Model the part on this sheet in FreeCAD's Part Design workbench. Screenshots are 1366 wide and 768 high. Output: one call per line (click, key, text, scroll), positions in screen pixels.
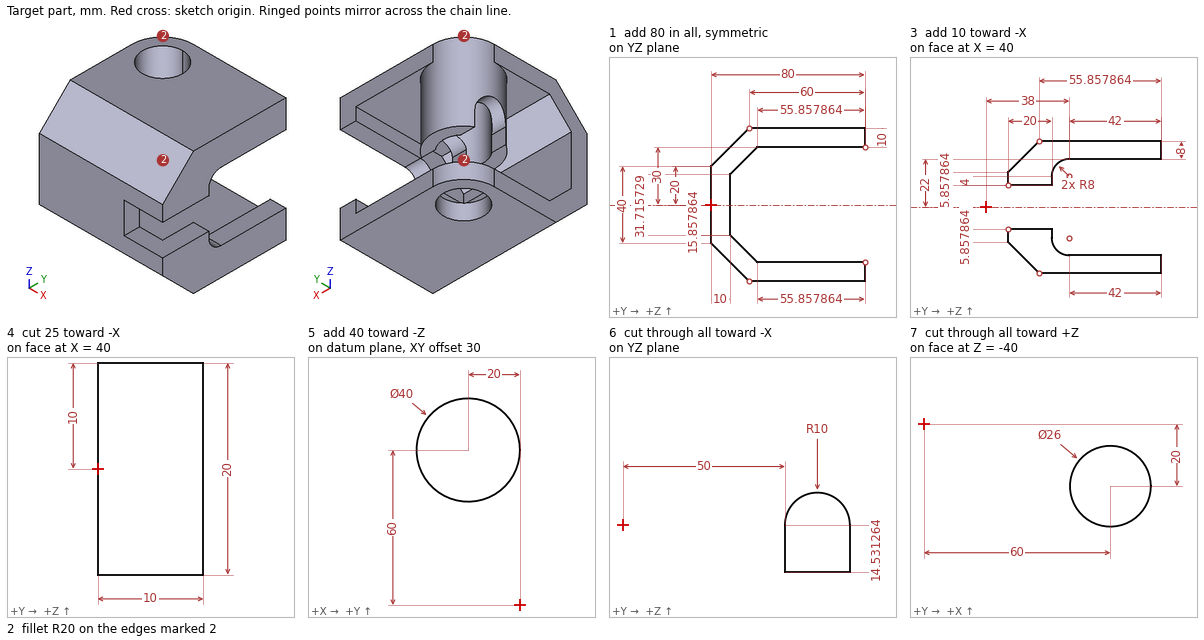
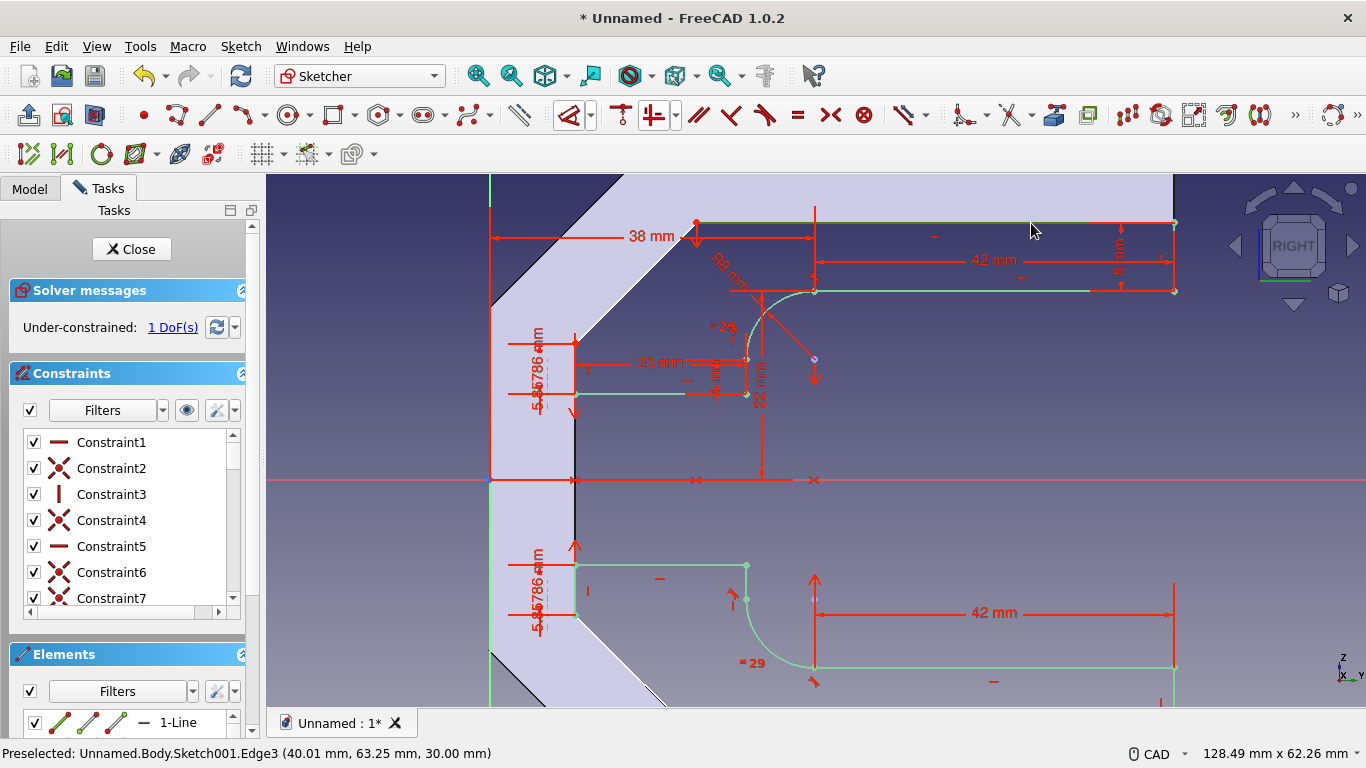
click(590, 116)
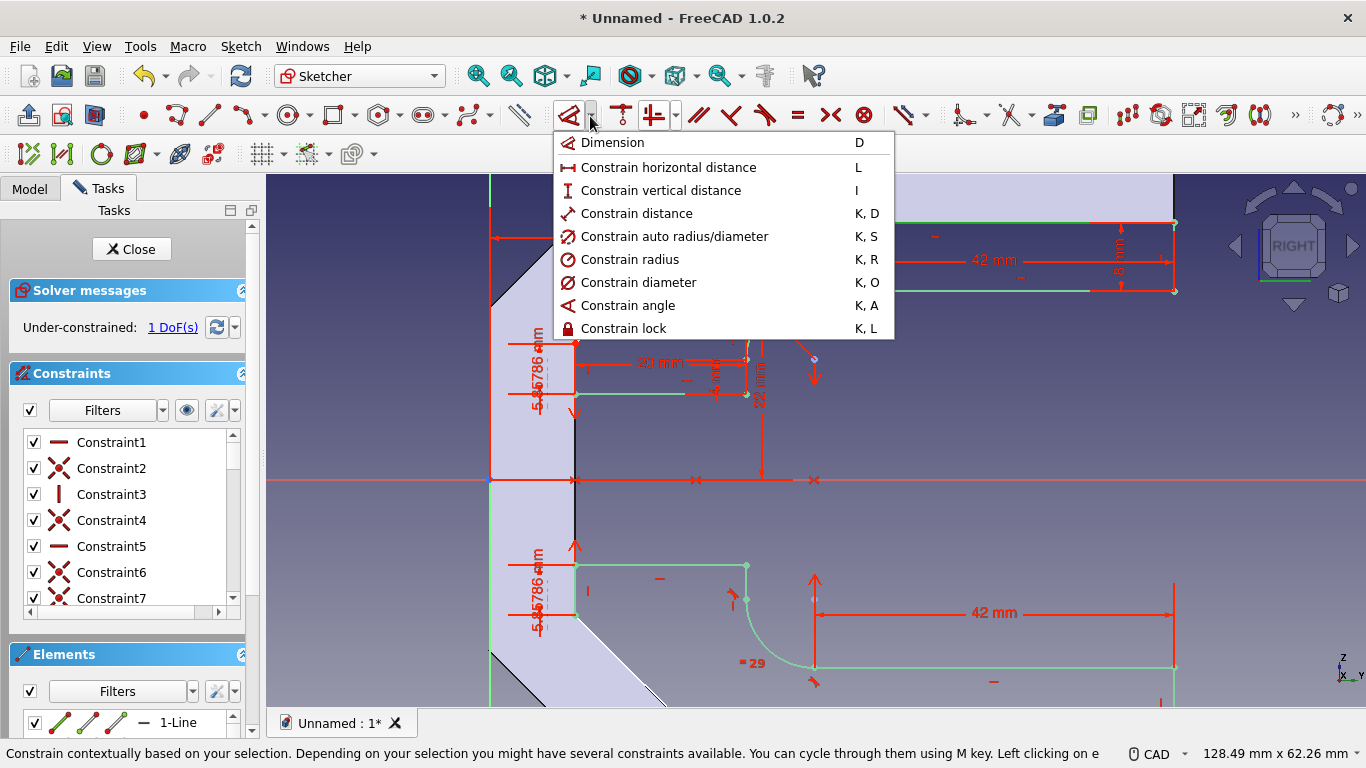
click(724, 168)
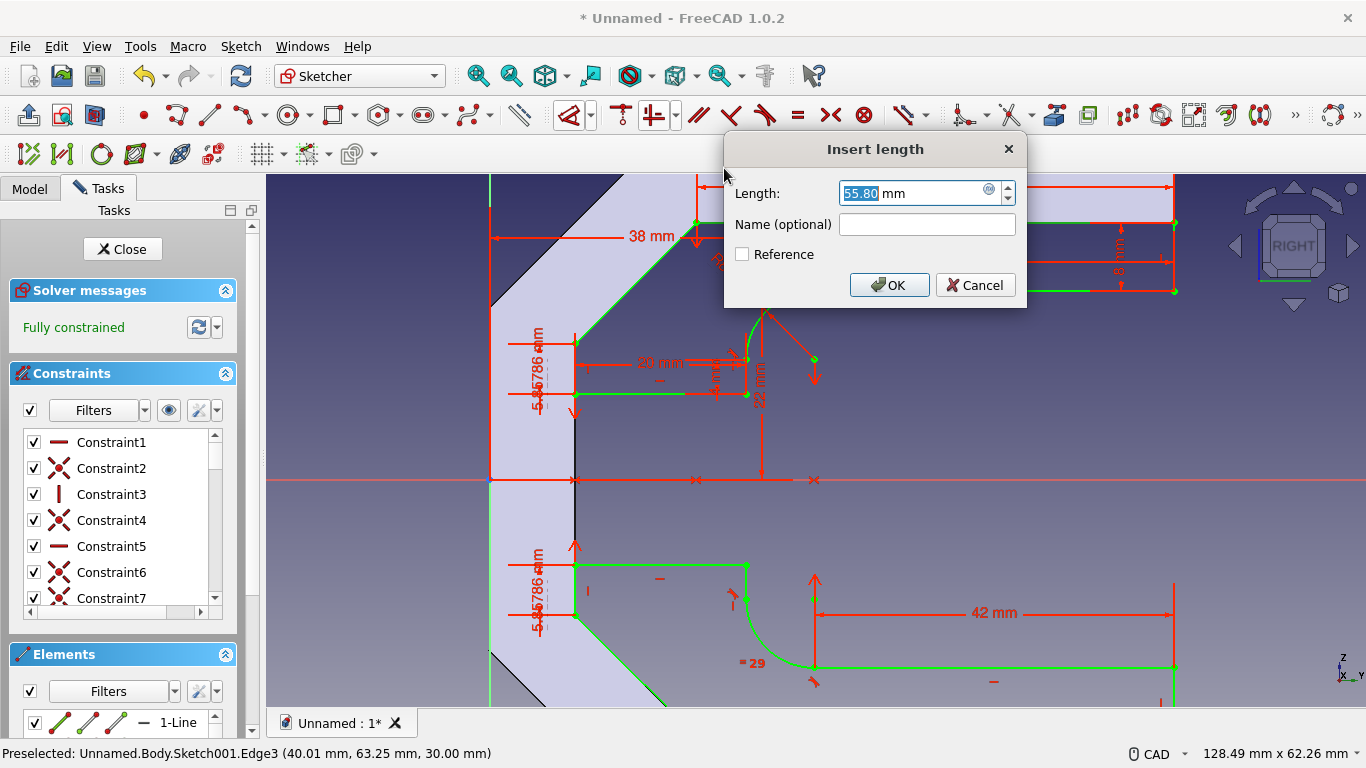
text(55.857864)
key(Return)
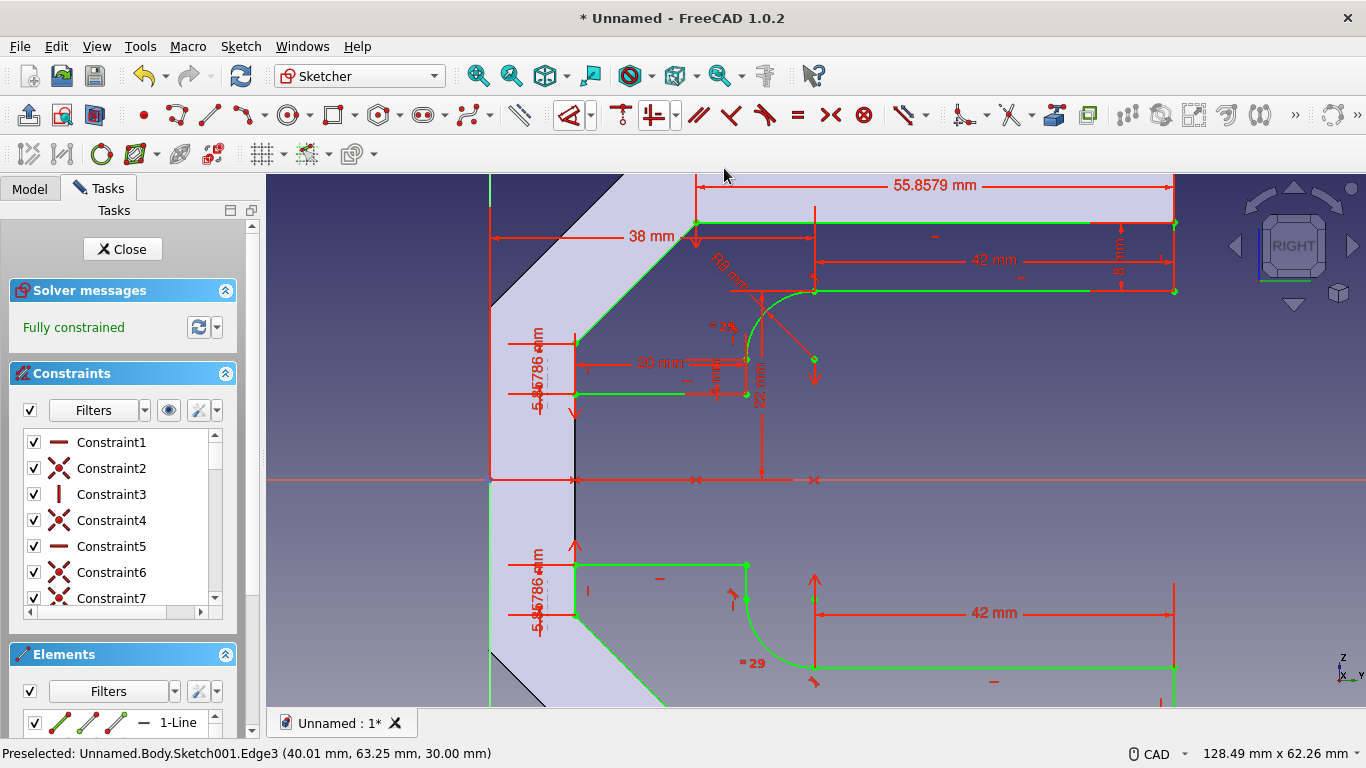
click(123, 249)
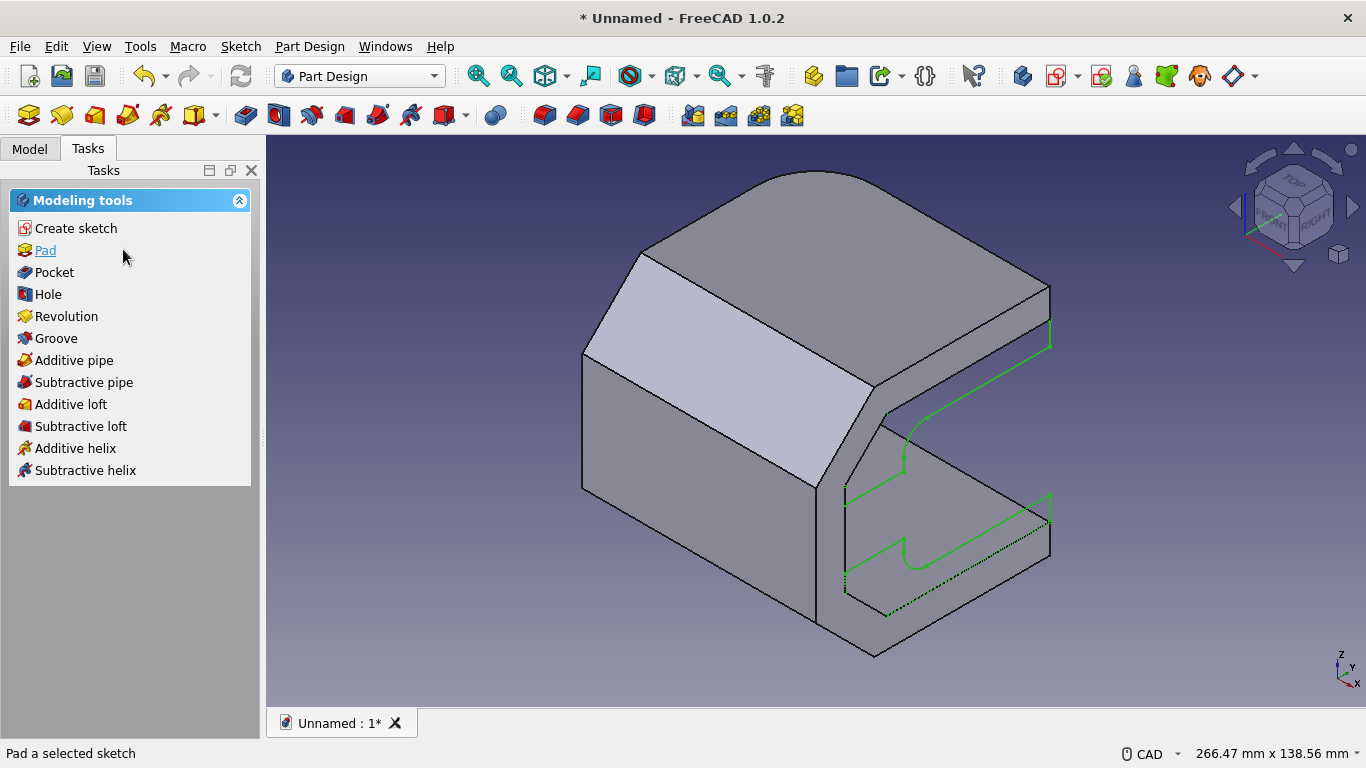
click(29, 116)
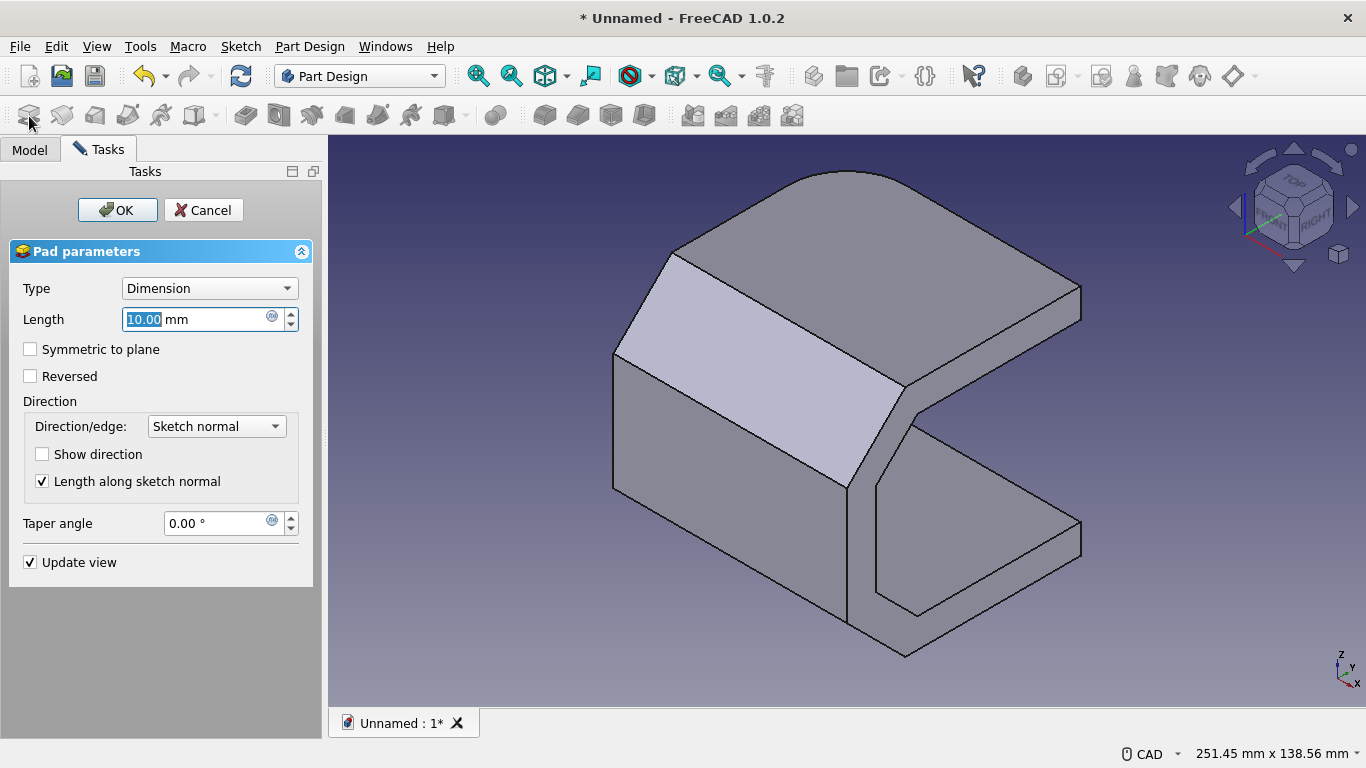
text(10)
key(Tab)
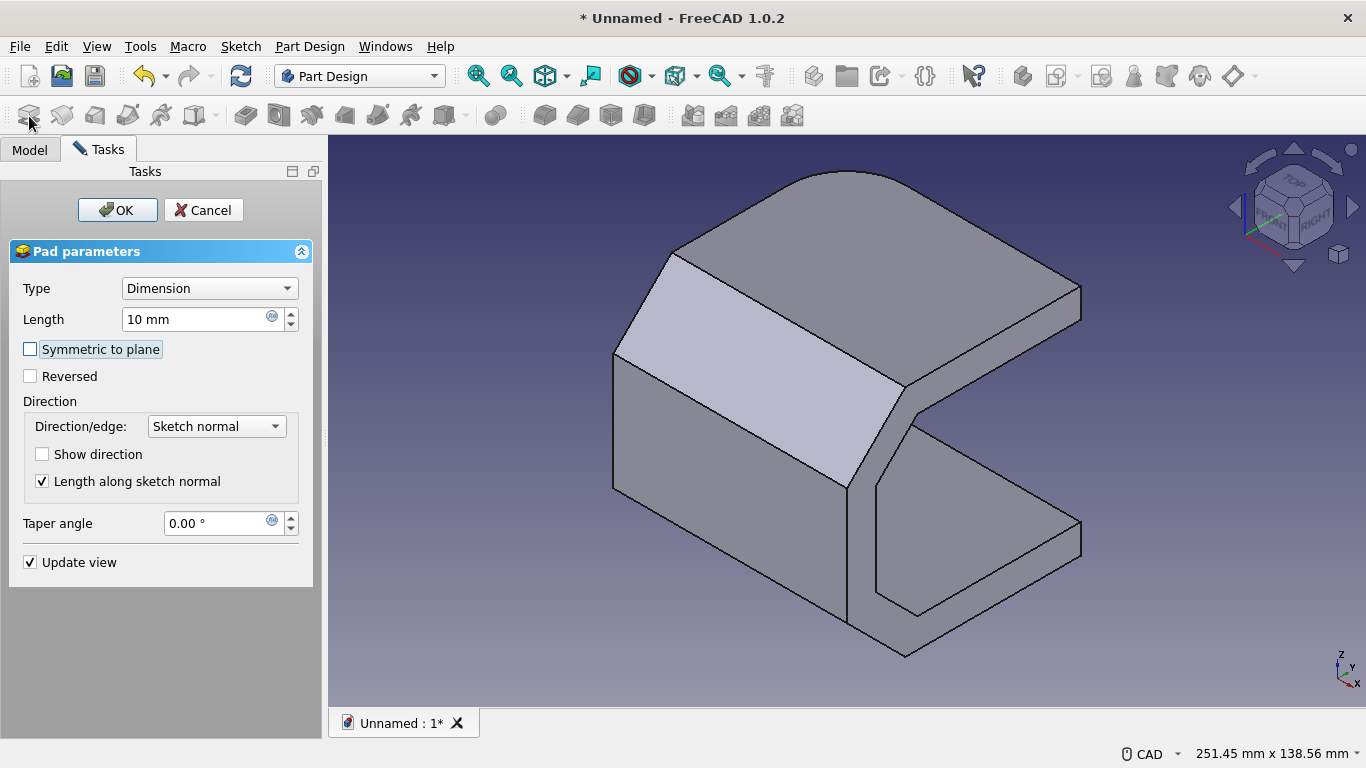
click(31, 376)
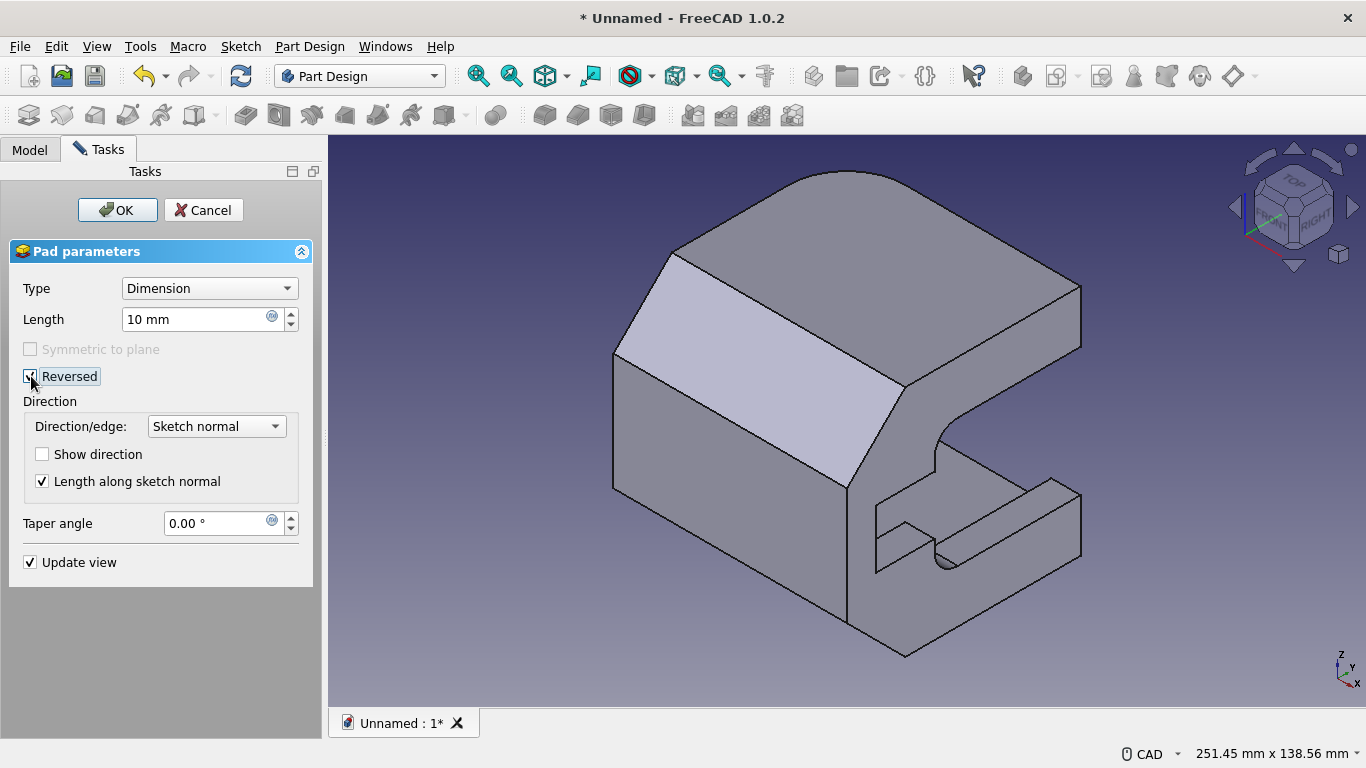
click(118, 210)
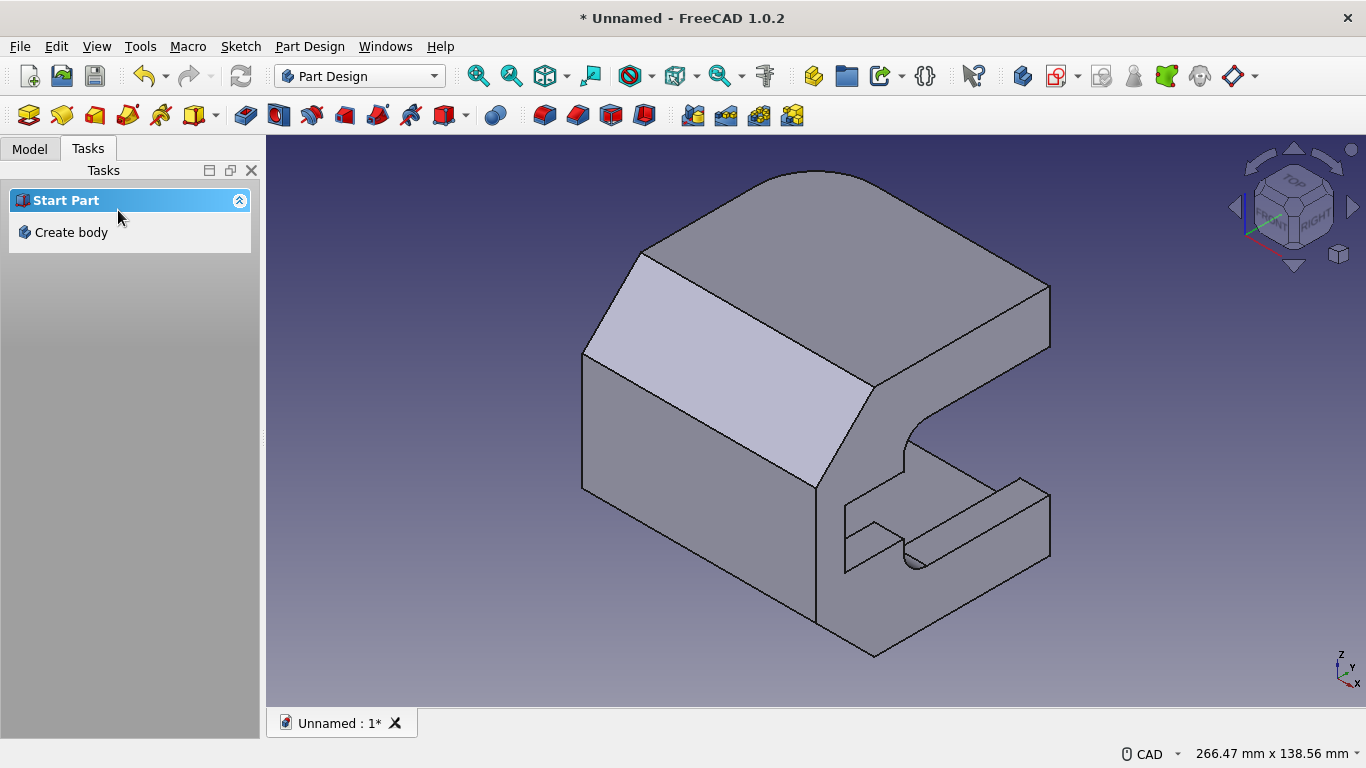
click(866, 449)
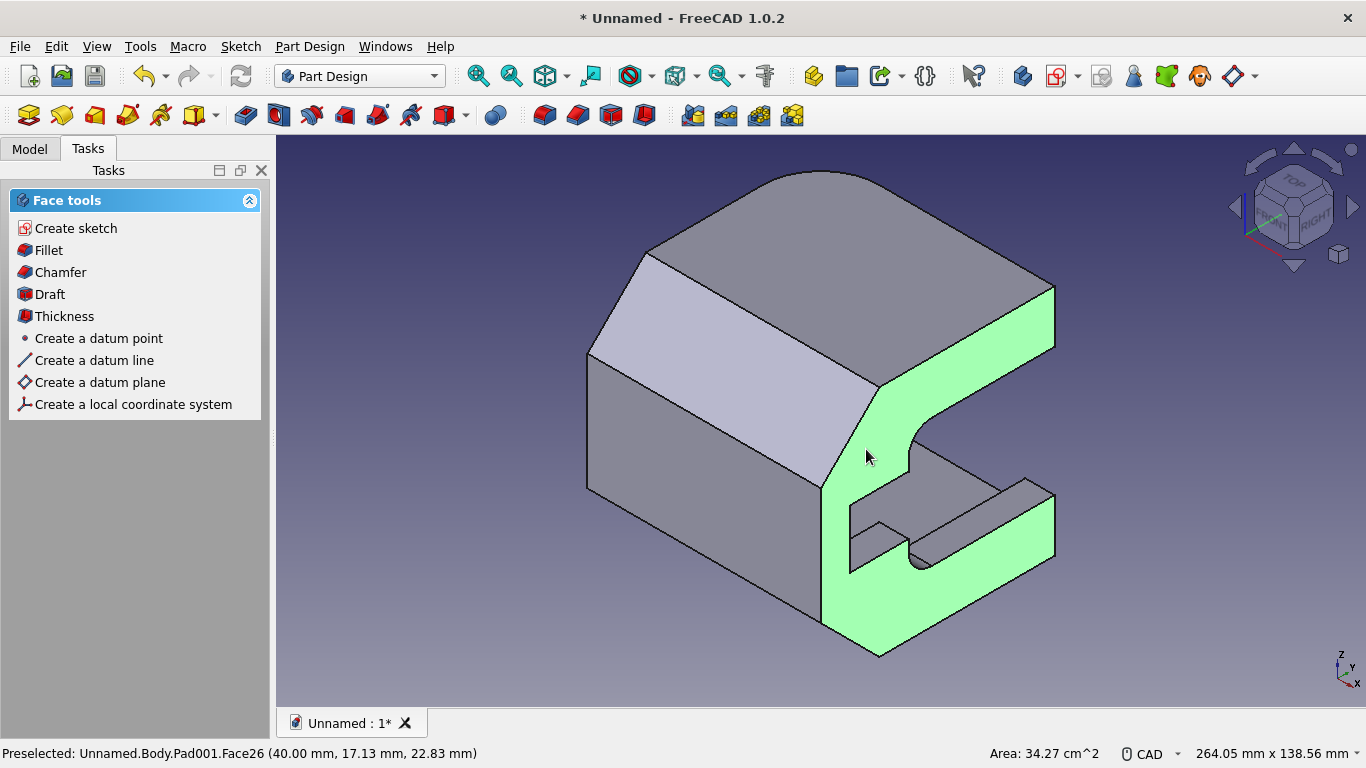
click(1056, 76)